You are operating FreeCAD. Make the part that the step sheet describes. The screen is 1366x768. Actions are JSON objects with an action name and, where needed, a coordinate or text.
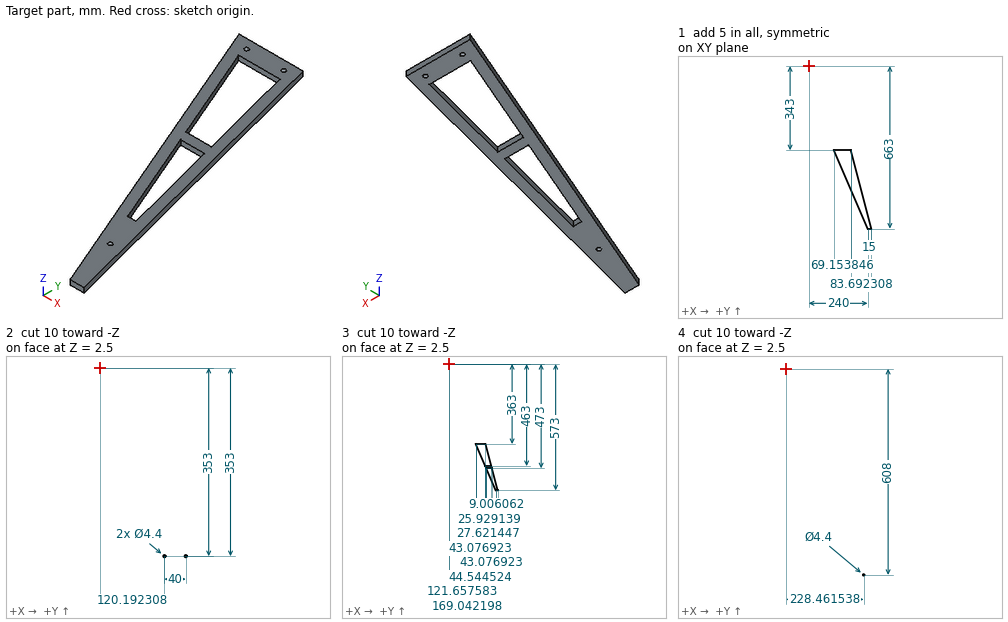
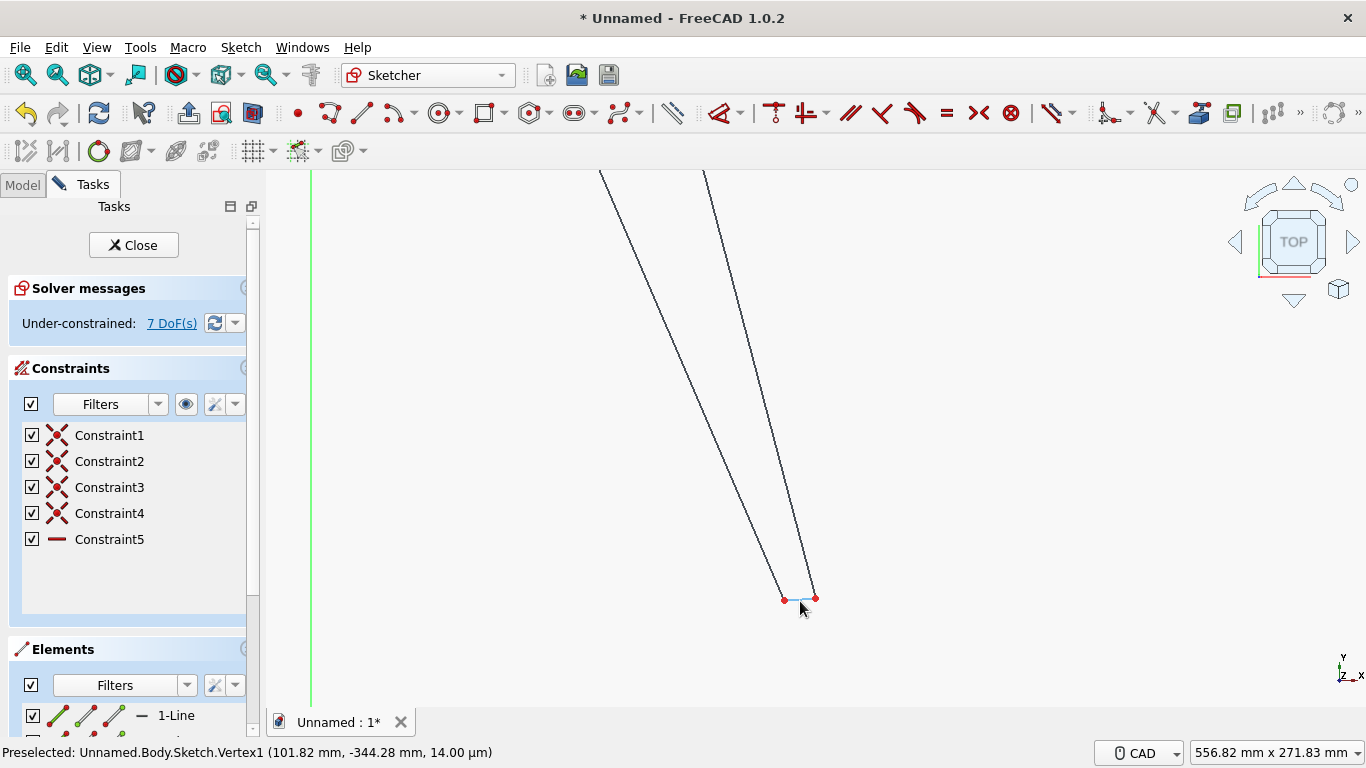
{"action": "left_click", "coordinate": [800, 600]}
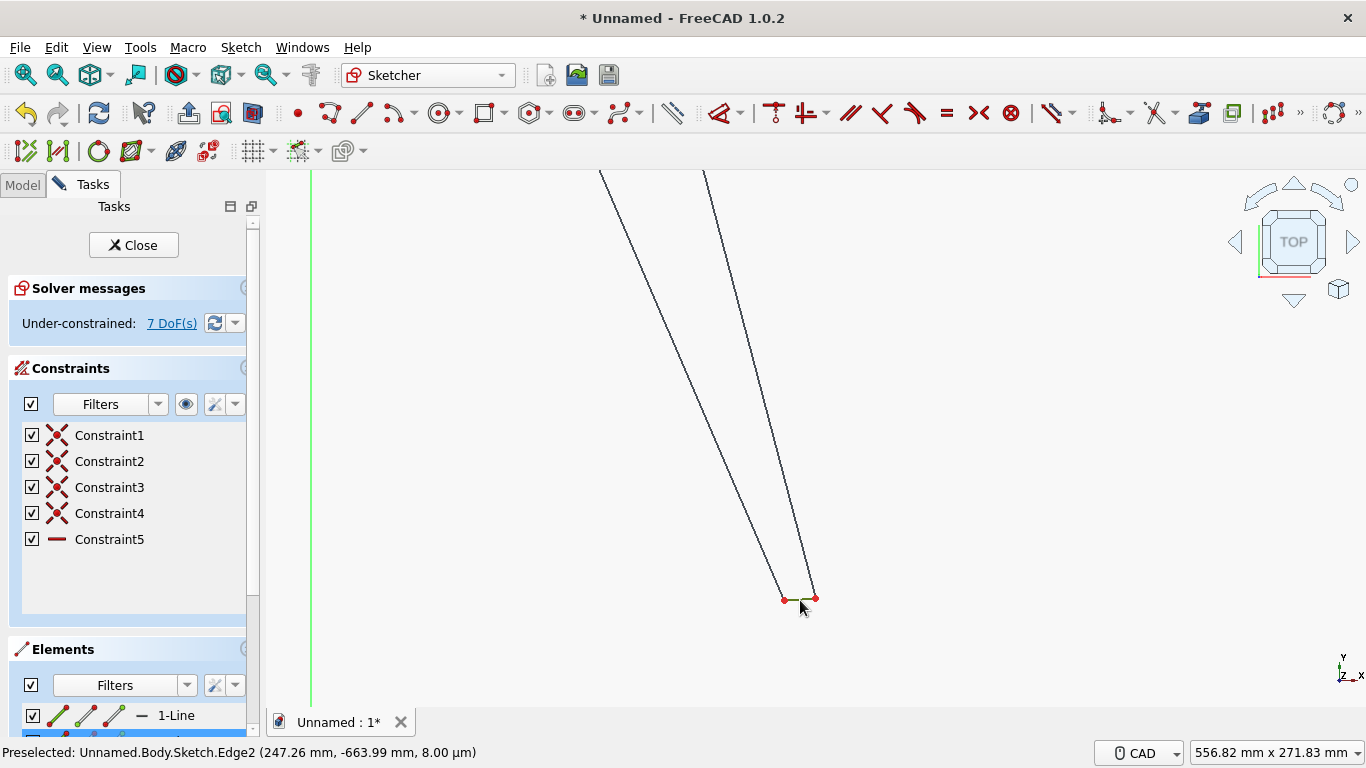
{"action": "key", "text": "h"}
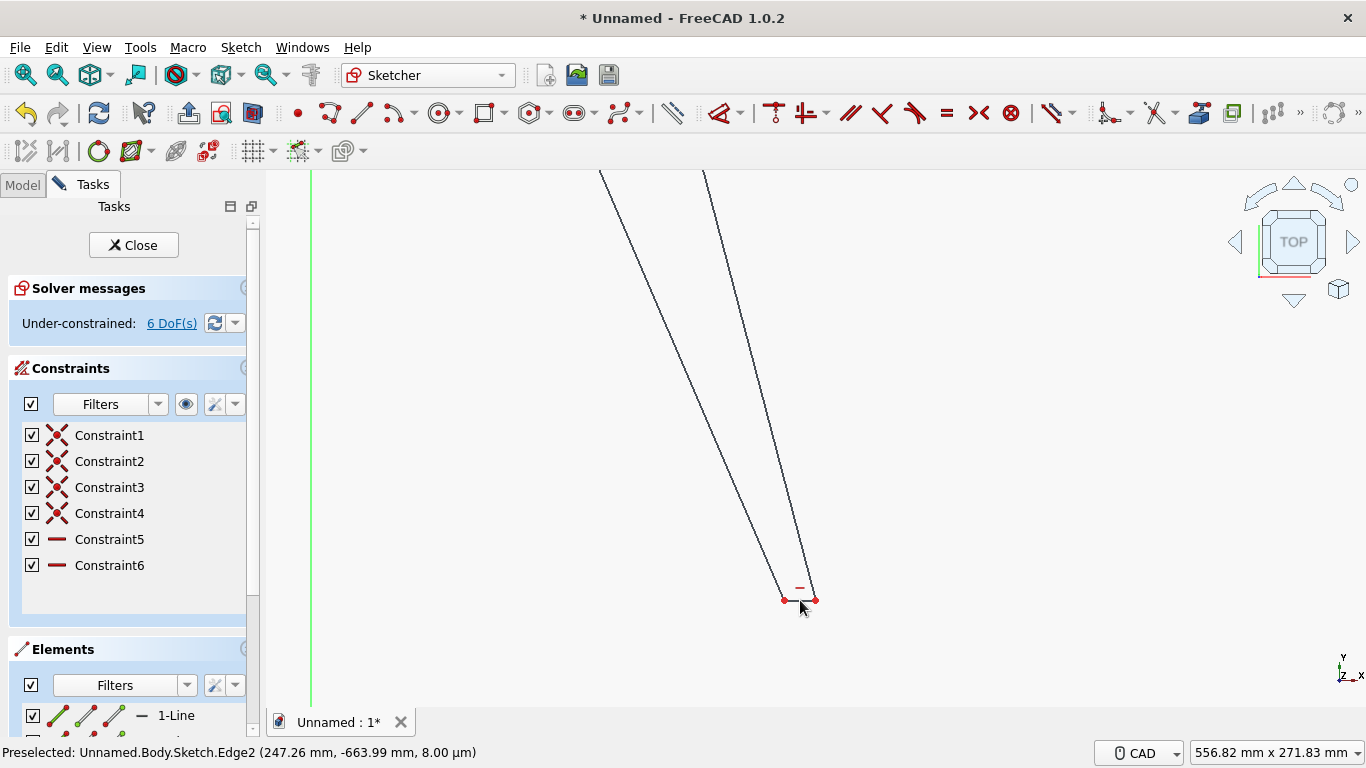
{"action": "key", "text": "d"}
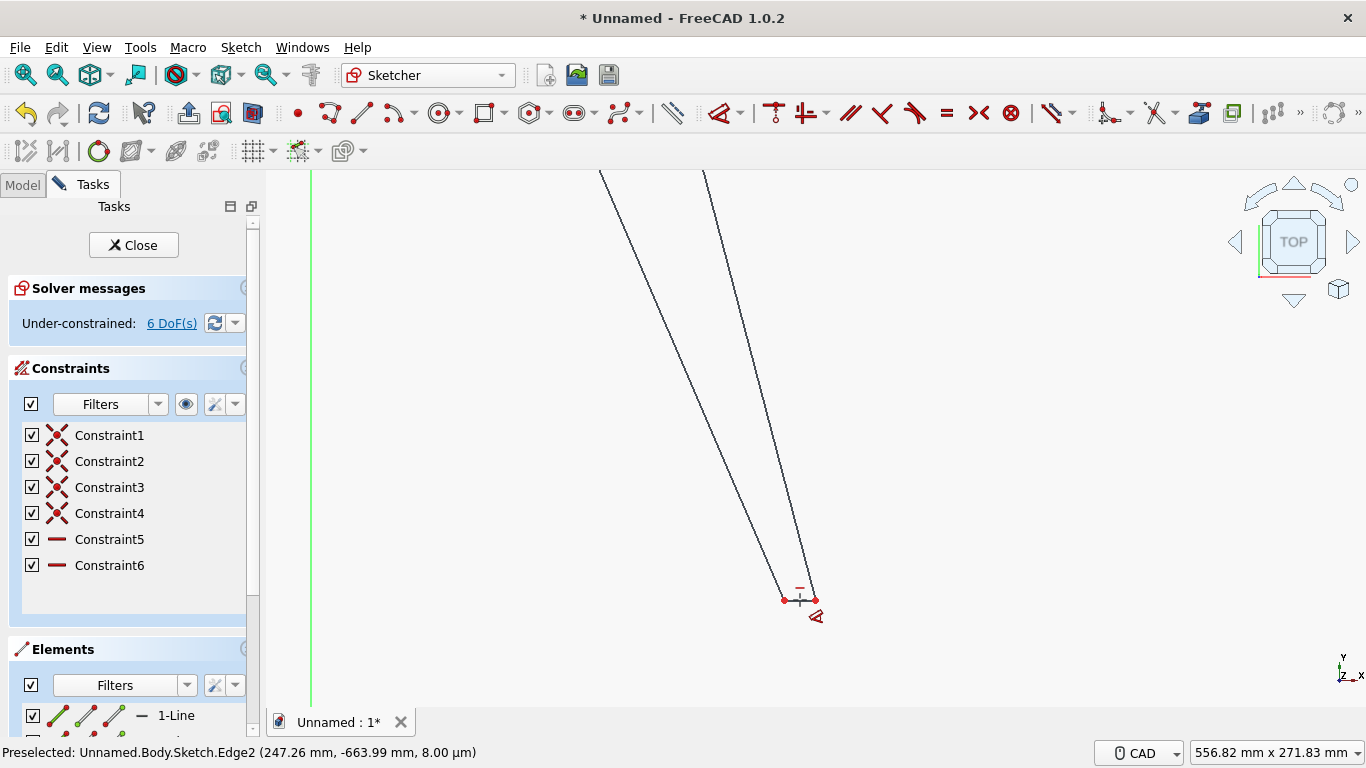
{"action": "scroll", "coordinate": [794, 601], "scroll_direction": "up", "scroll_amount": 2}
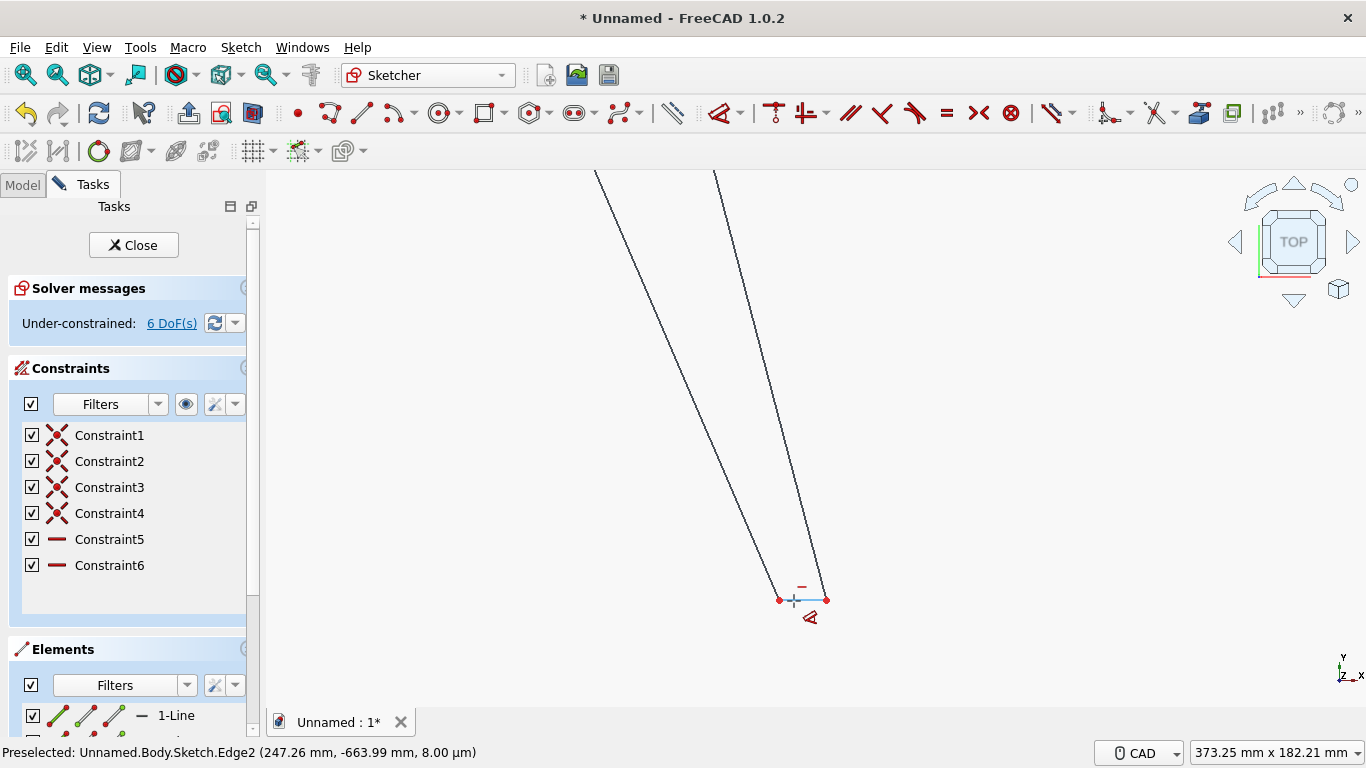
{"action": "left_click", "coordinate": [793, 600]}
{"action": "left_click", "coordinate": [803, 634]}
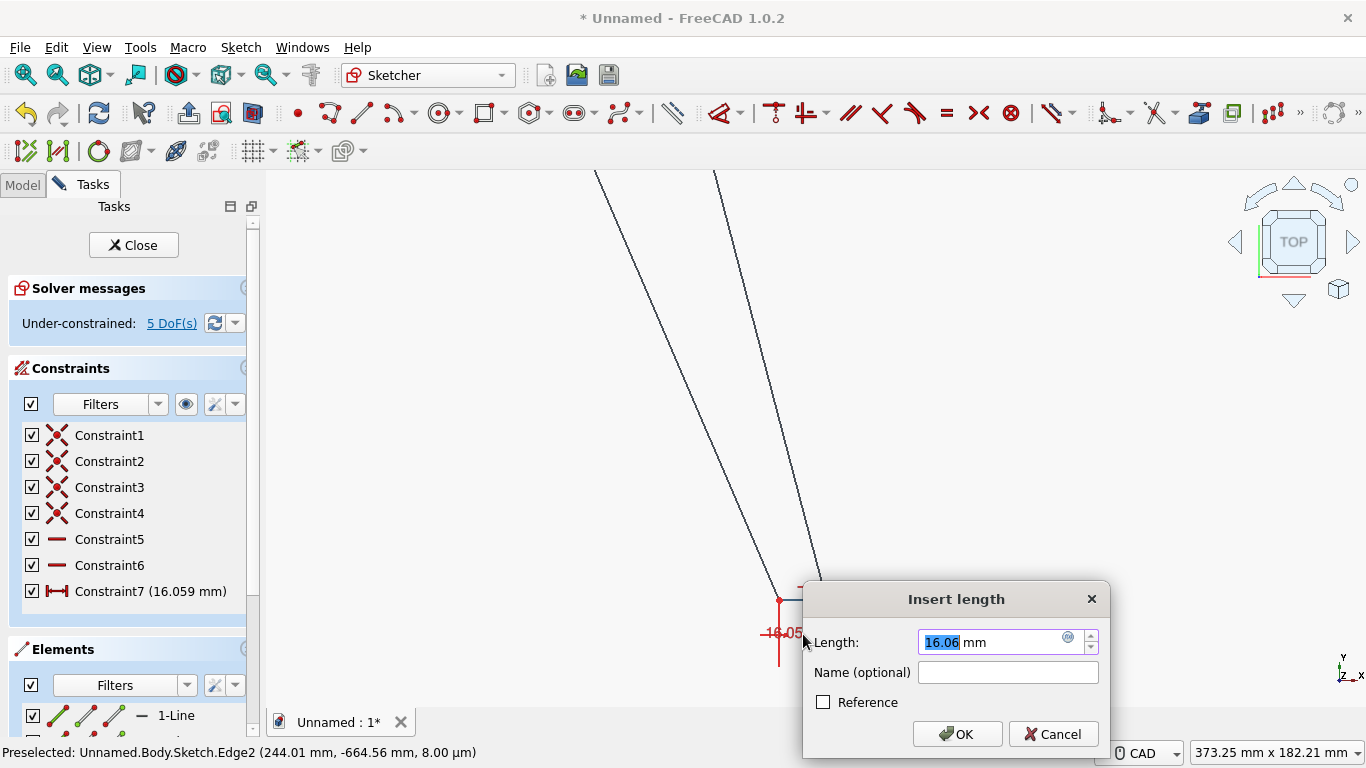
{"action": "type", "text": "15"}
{"action": "key", "text": "Return"}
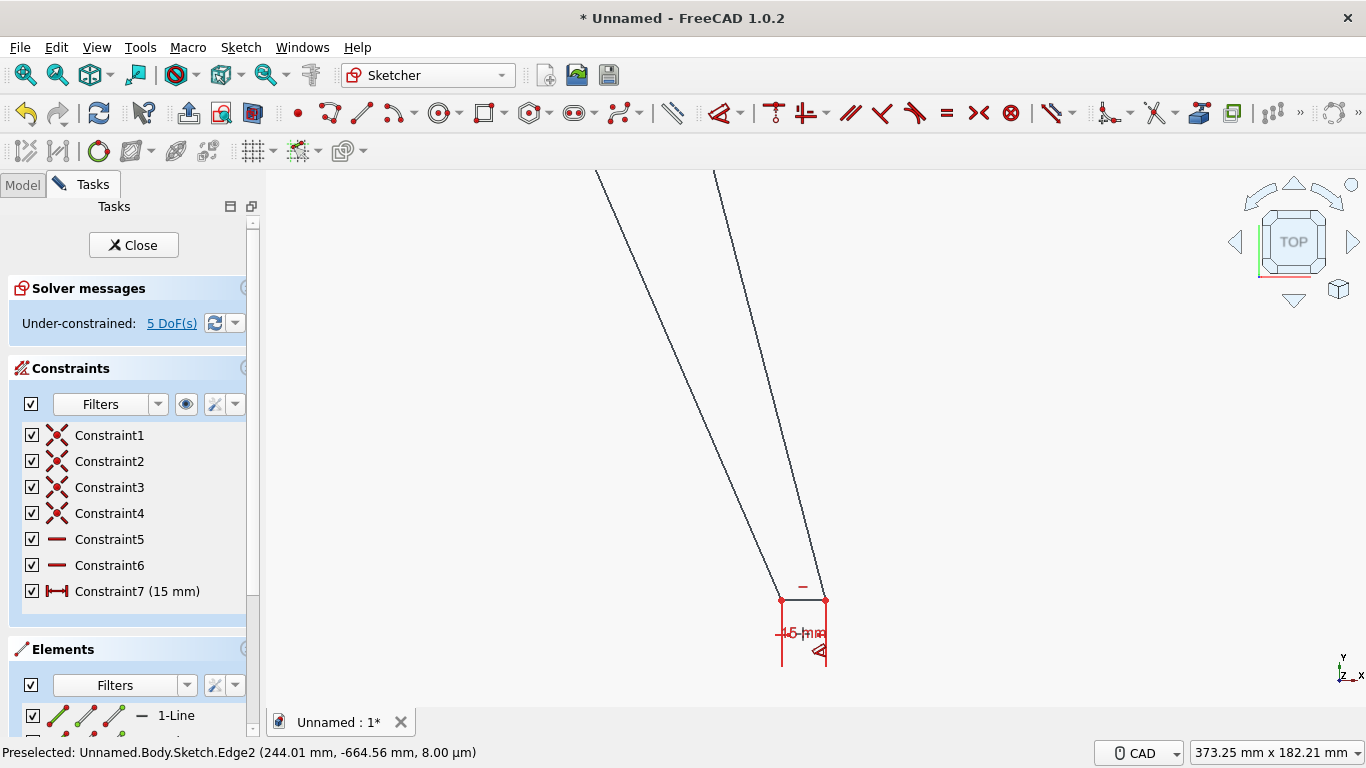
{"action": "scroll", "coordinate": [806, 601], "scroll_direction": "down", "scroll_amount": 9}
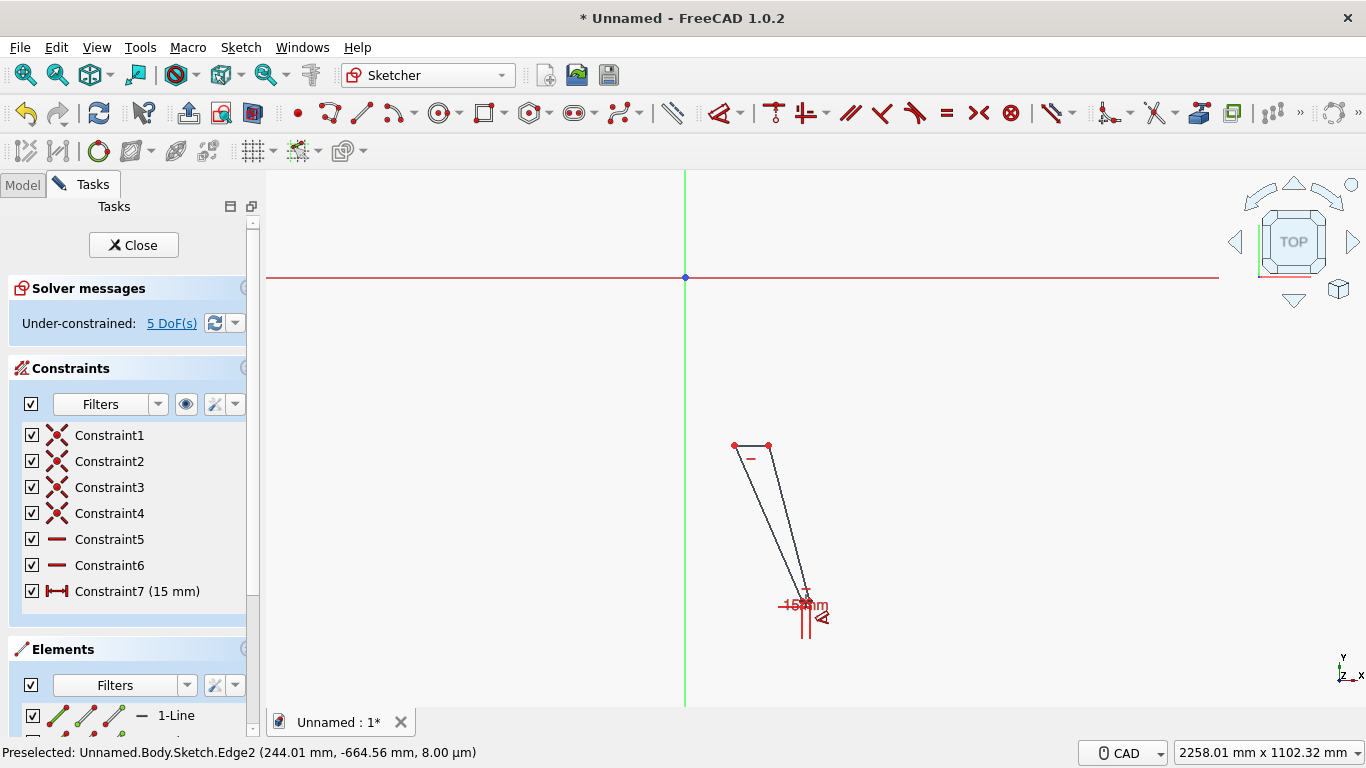
{"action": "left_click", "coordinate": [735, 446]}
{"action": "left_click", "coordinate": [651, 362]}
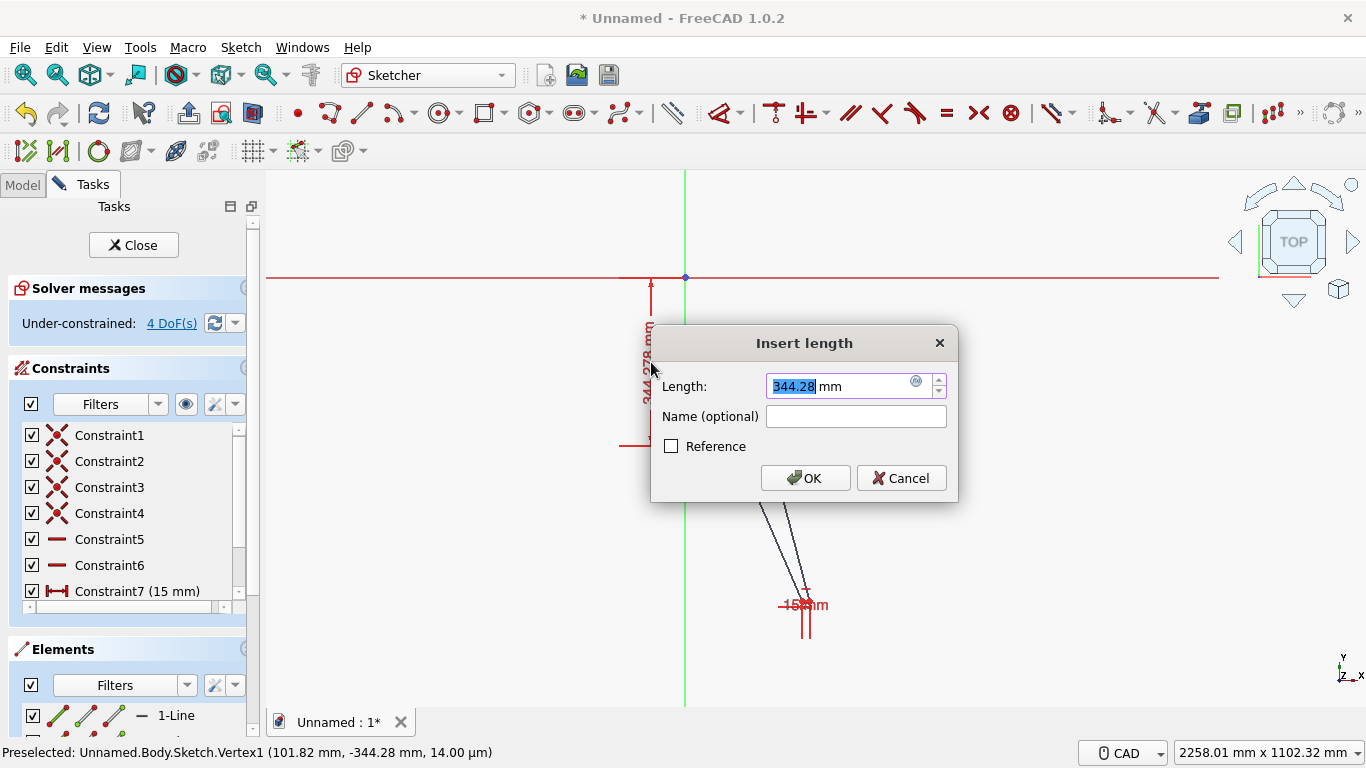
{"action": "type", "text": "343"}
{"action": "key", "text": "Return"}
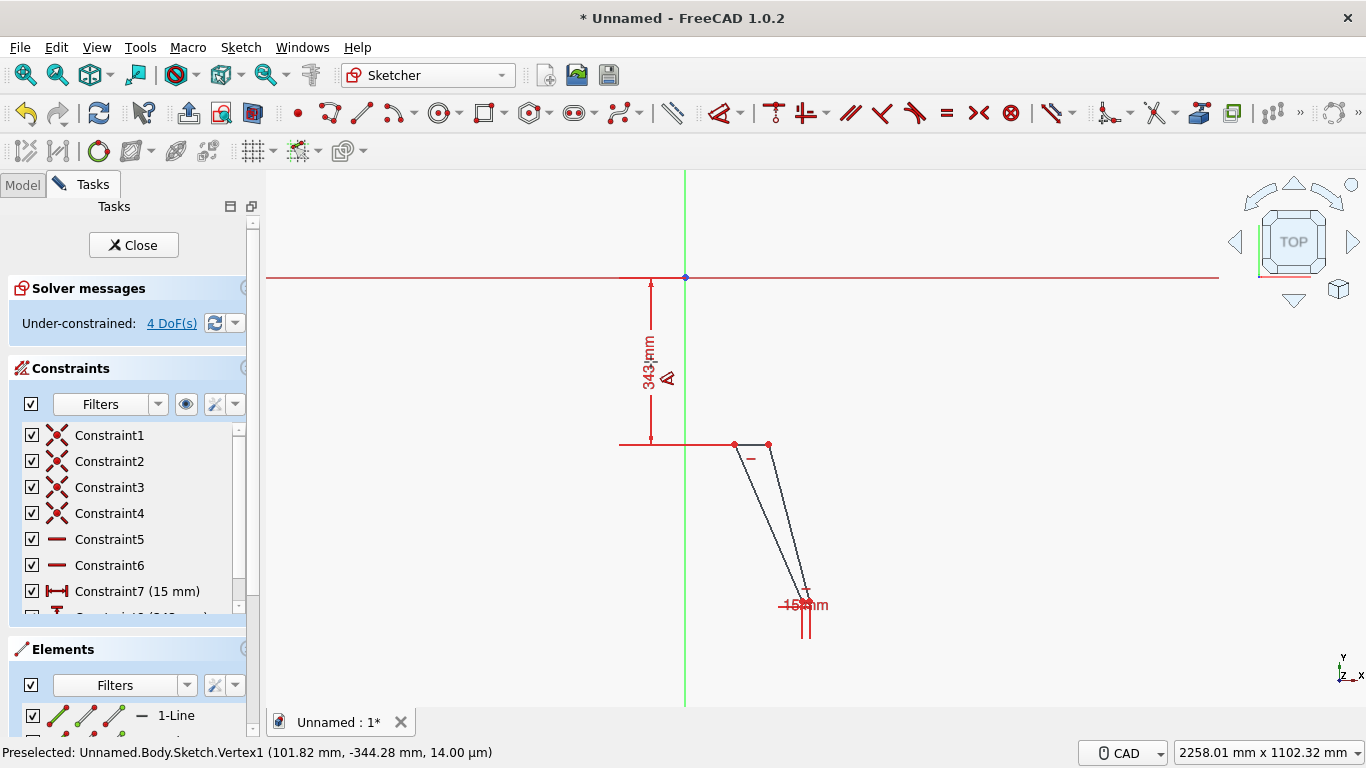
{"action": "scroll", "coordinate": [802, 602], "scroll_direction": "up", "scroll_amount": 3}